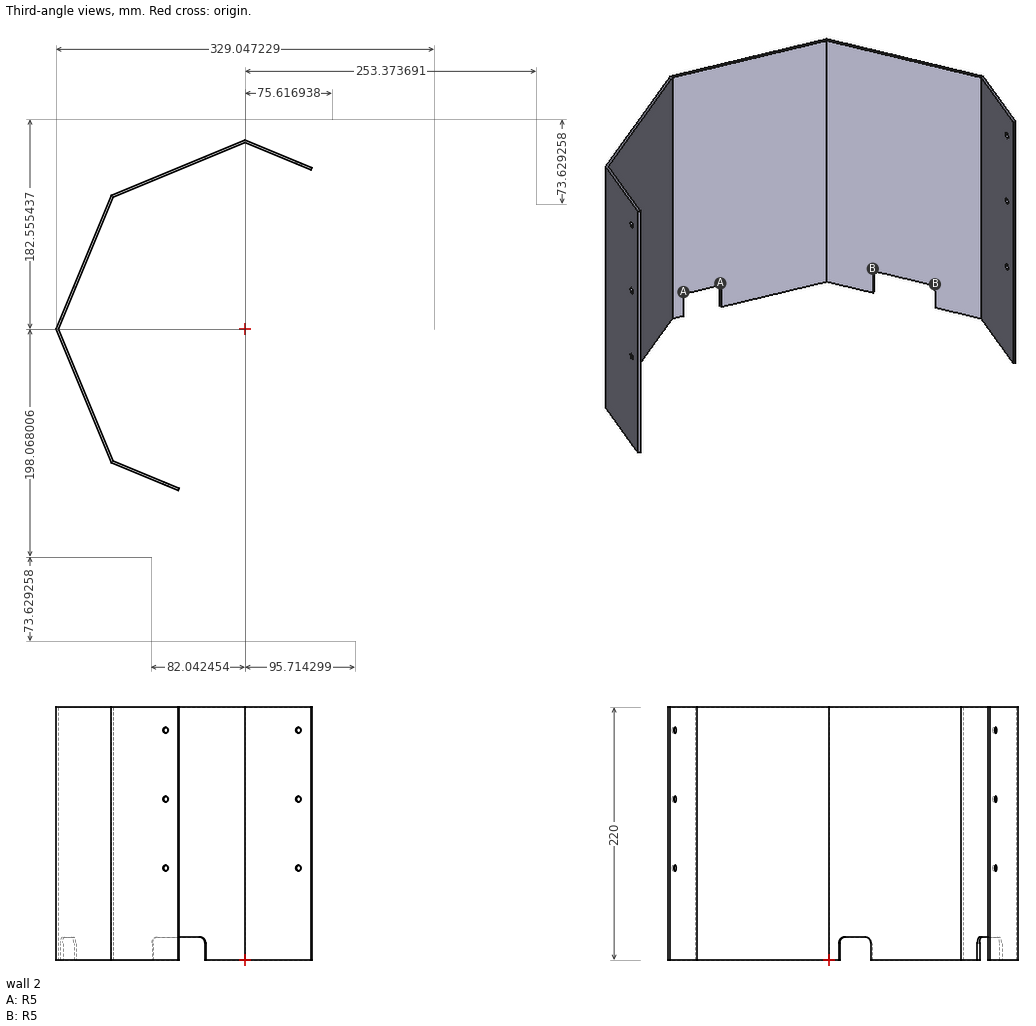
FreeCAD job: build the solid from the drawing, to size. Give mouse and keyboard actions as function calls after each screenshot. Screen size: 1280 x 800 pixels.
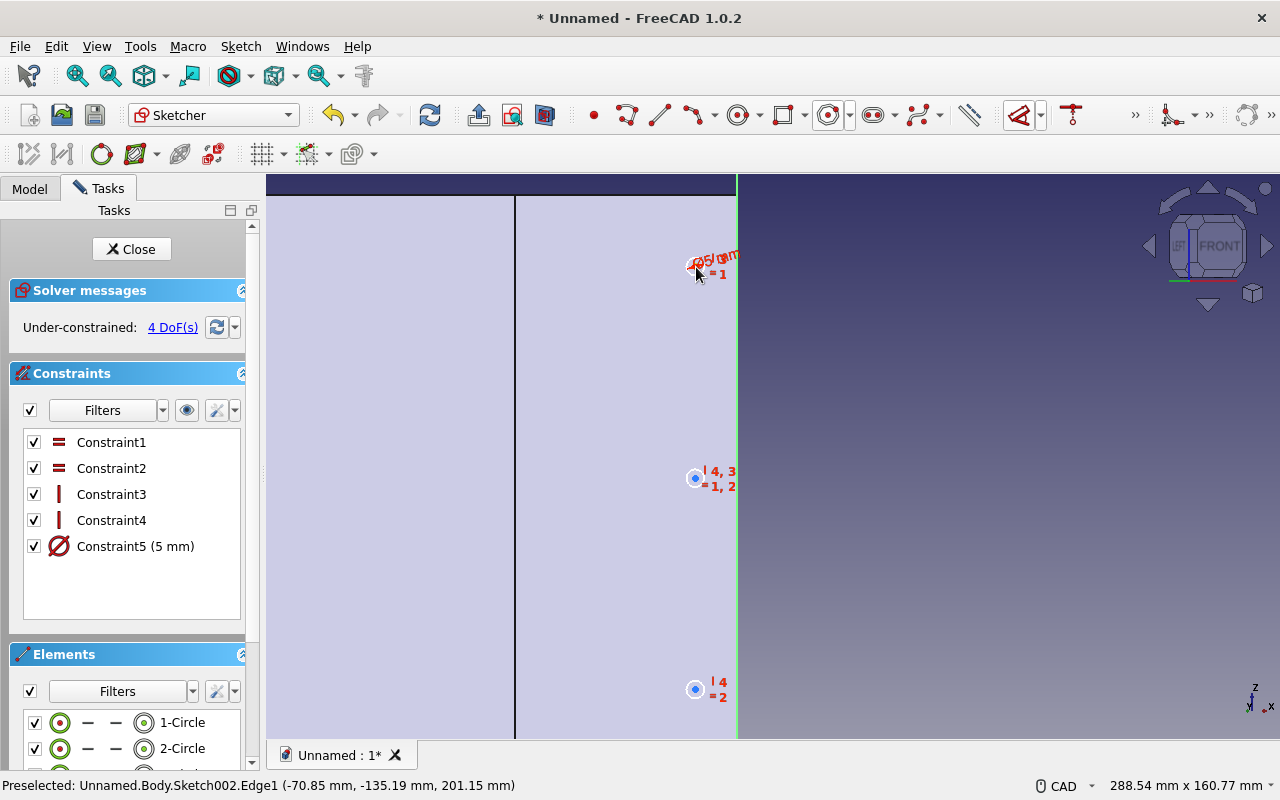
click(695, 267)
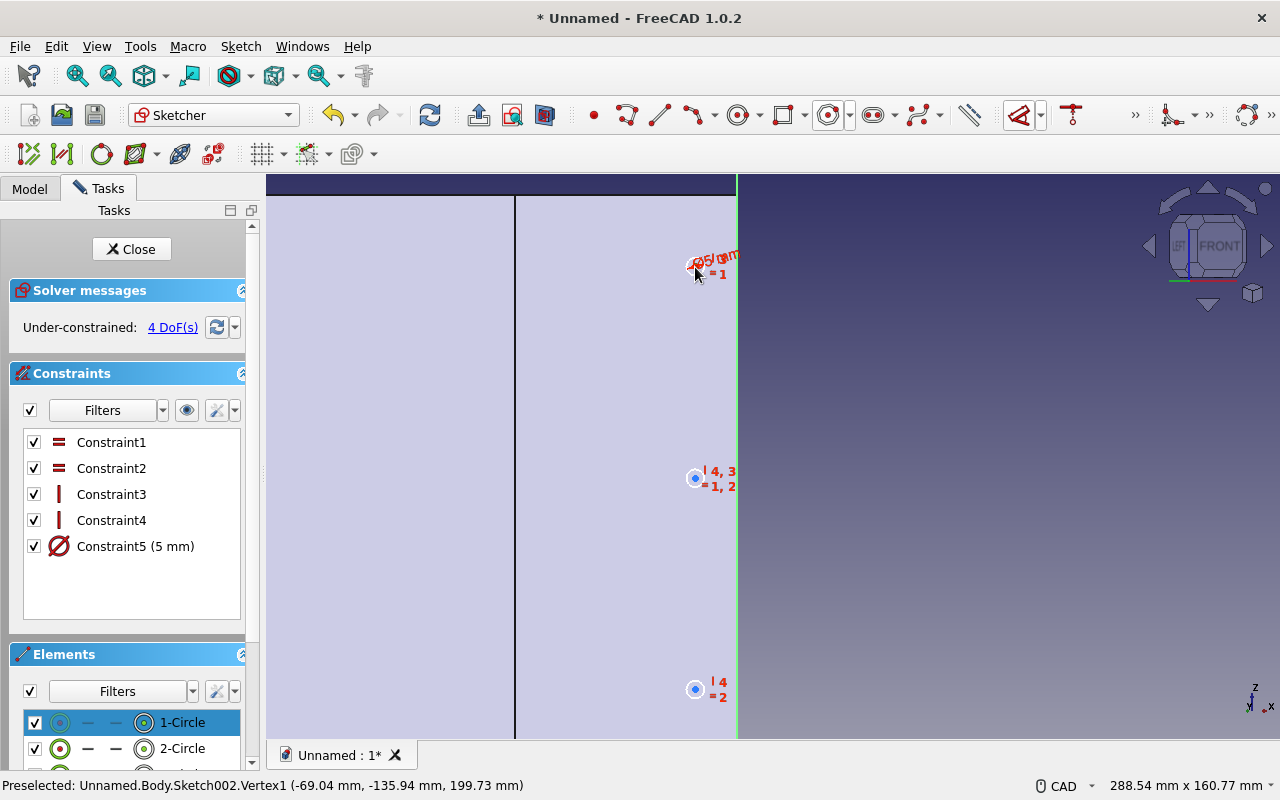
click(1040, 116)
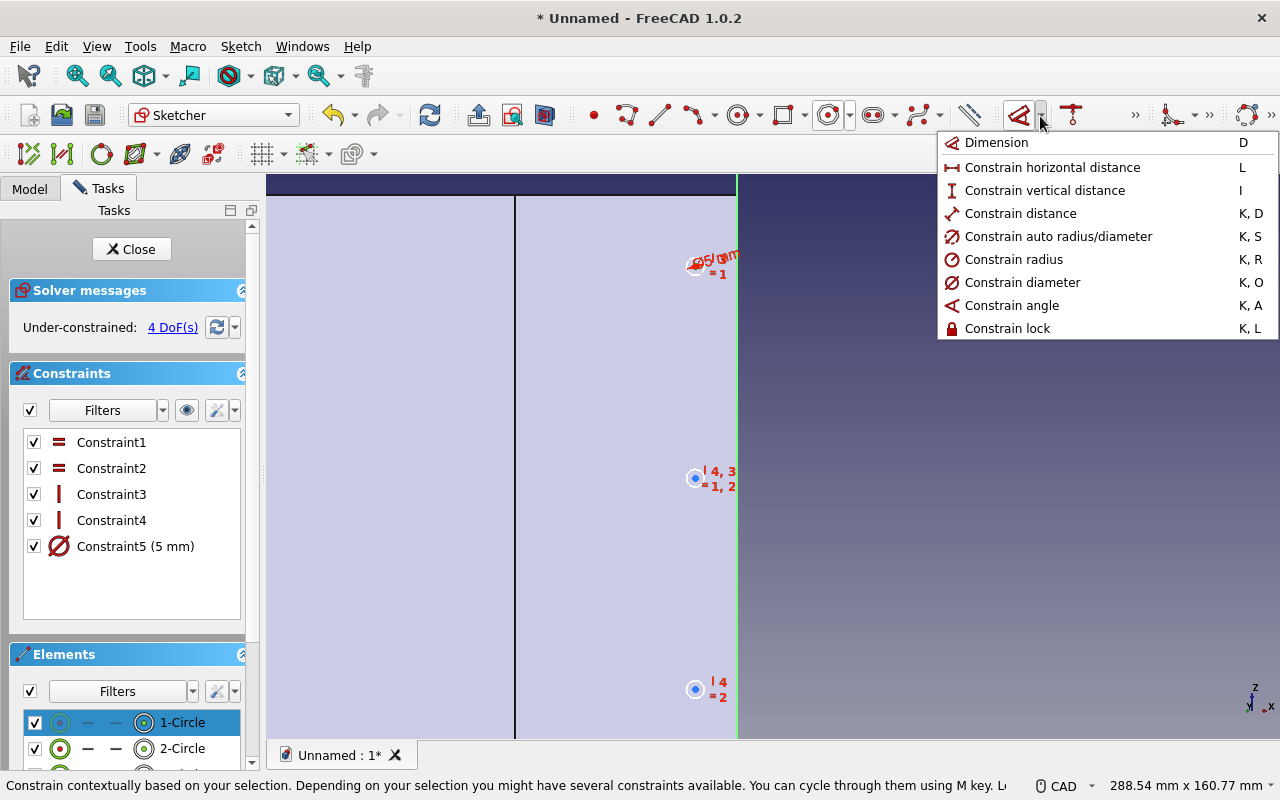
click(1108, 168)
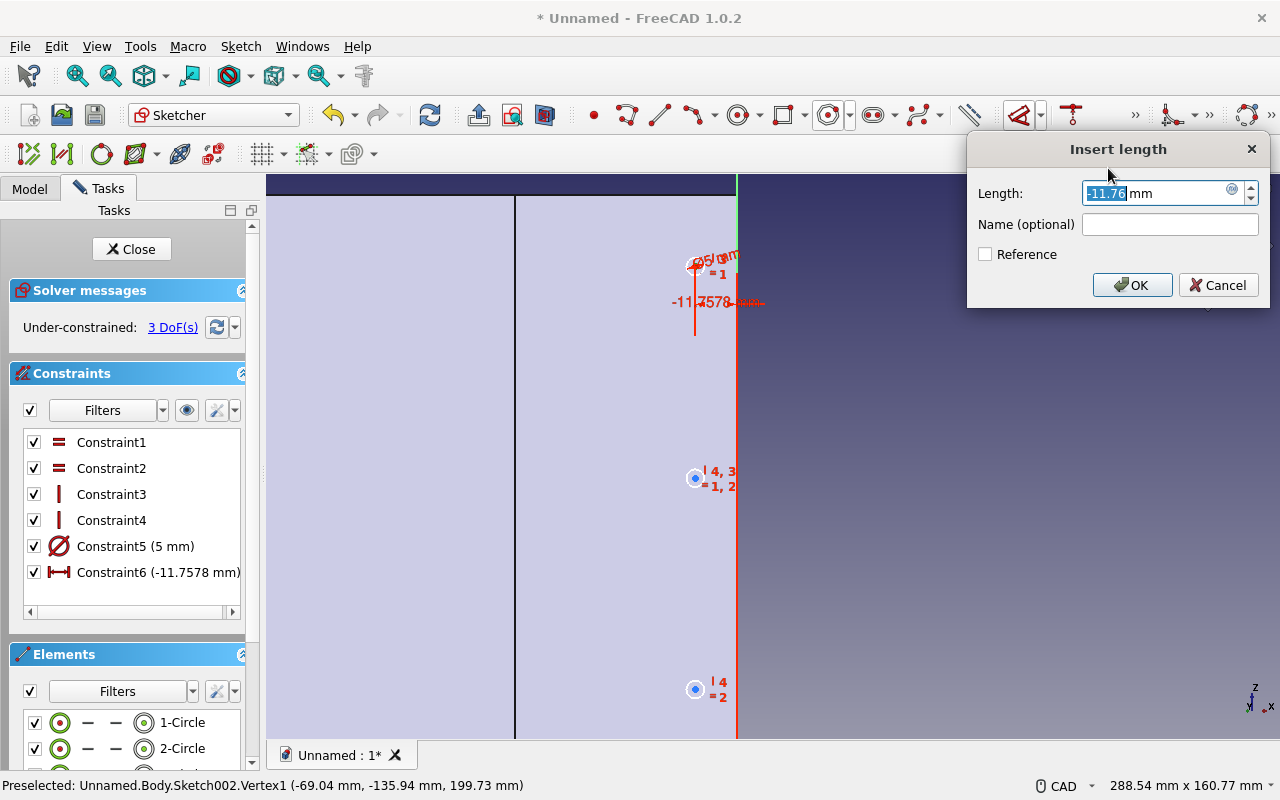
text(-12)
key(Return)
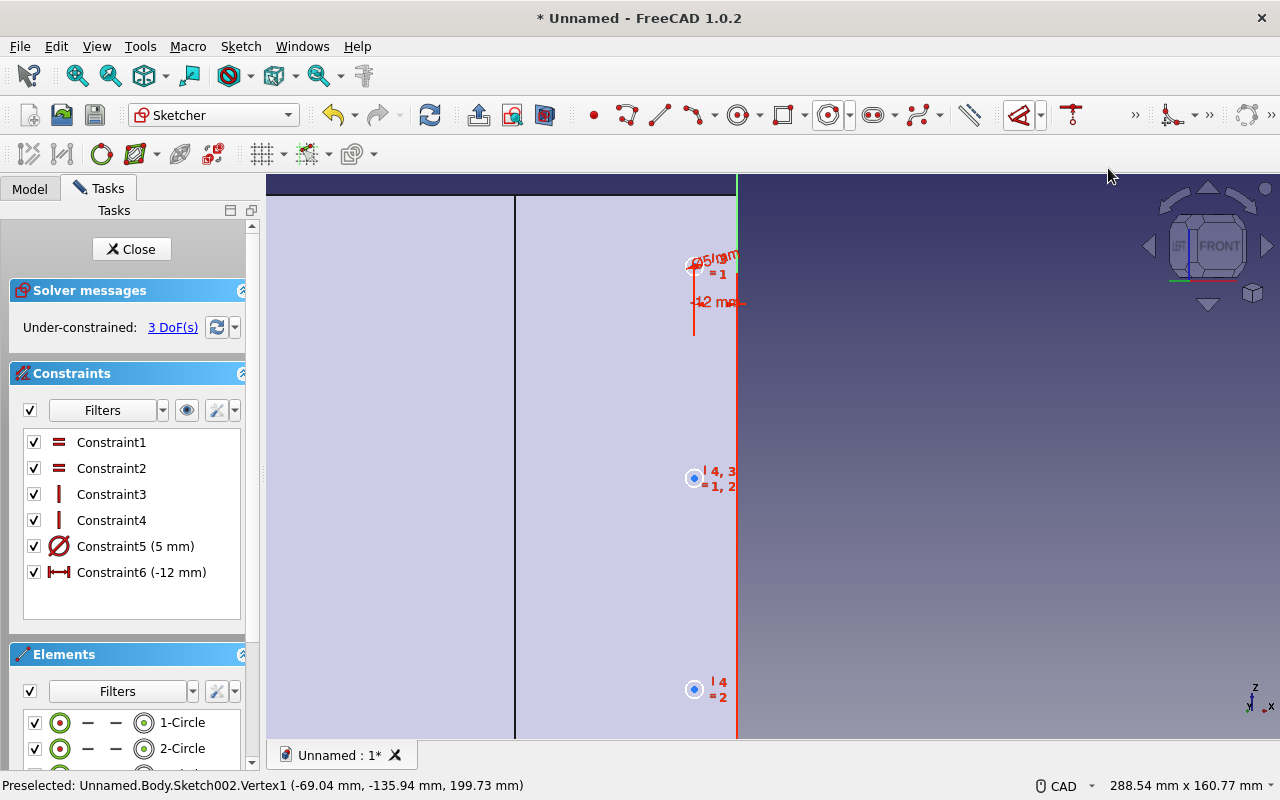
click(694, 690)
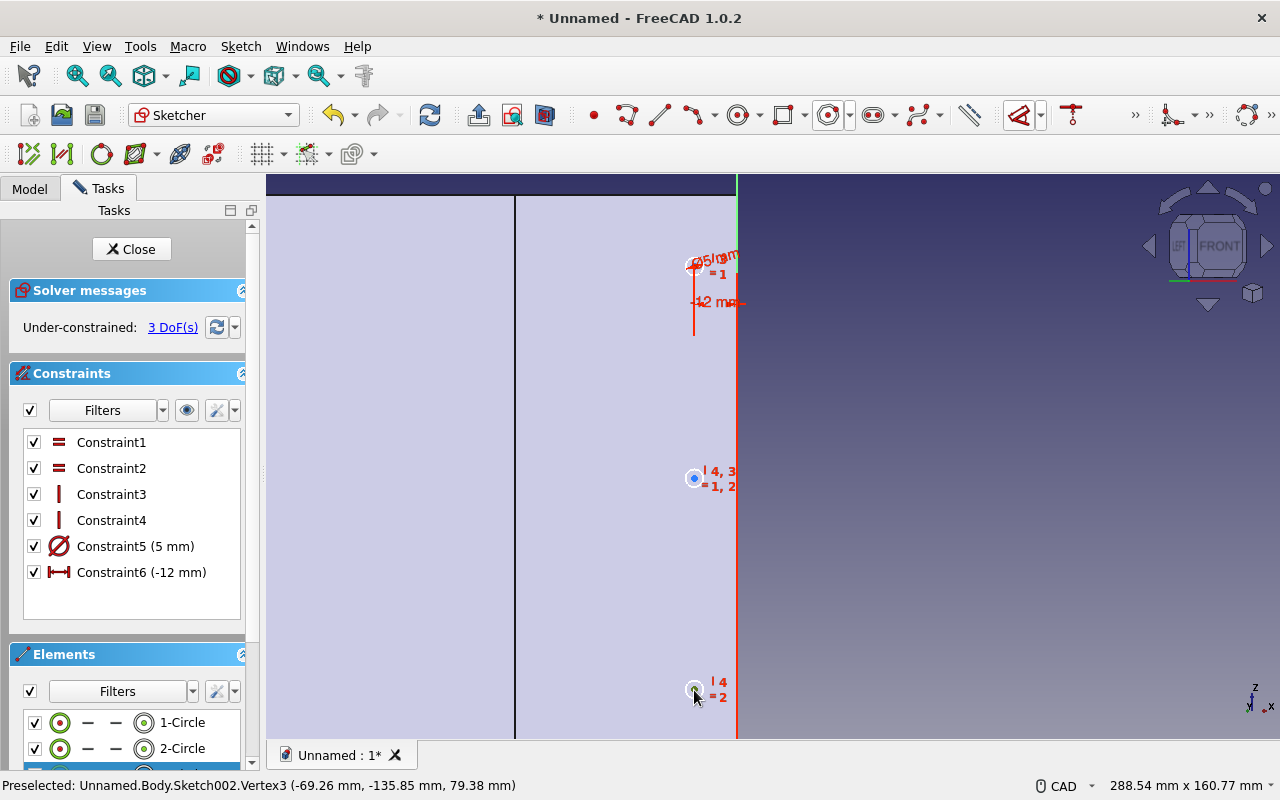
click(1040, 116)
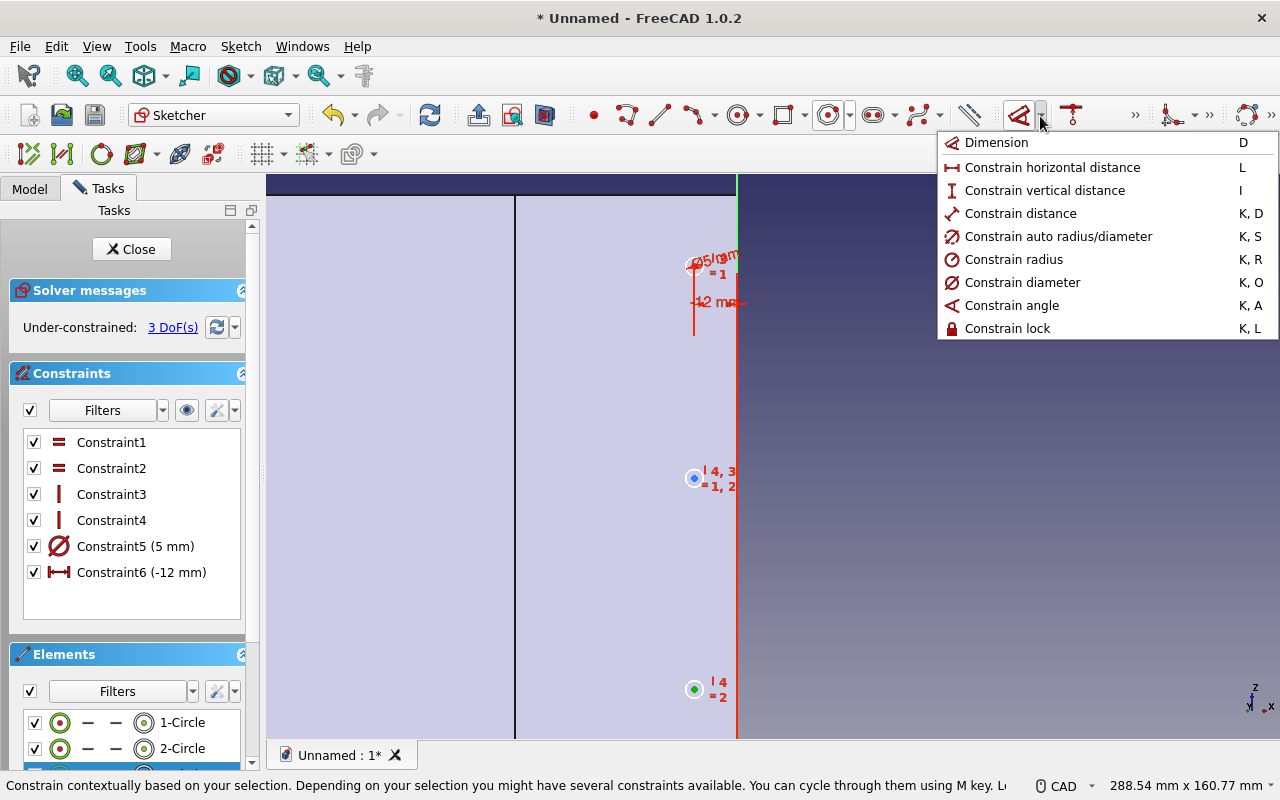
click(1108, 190)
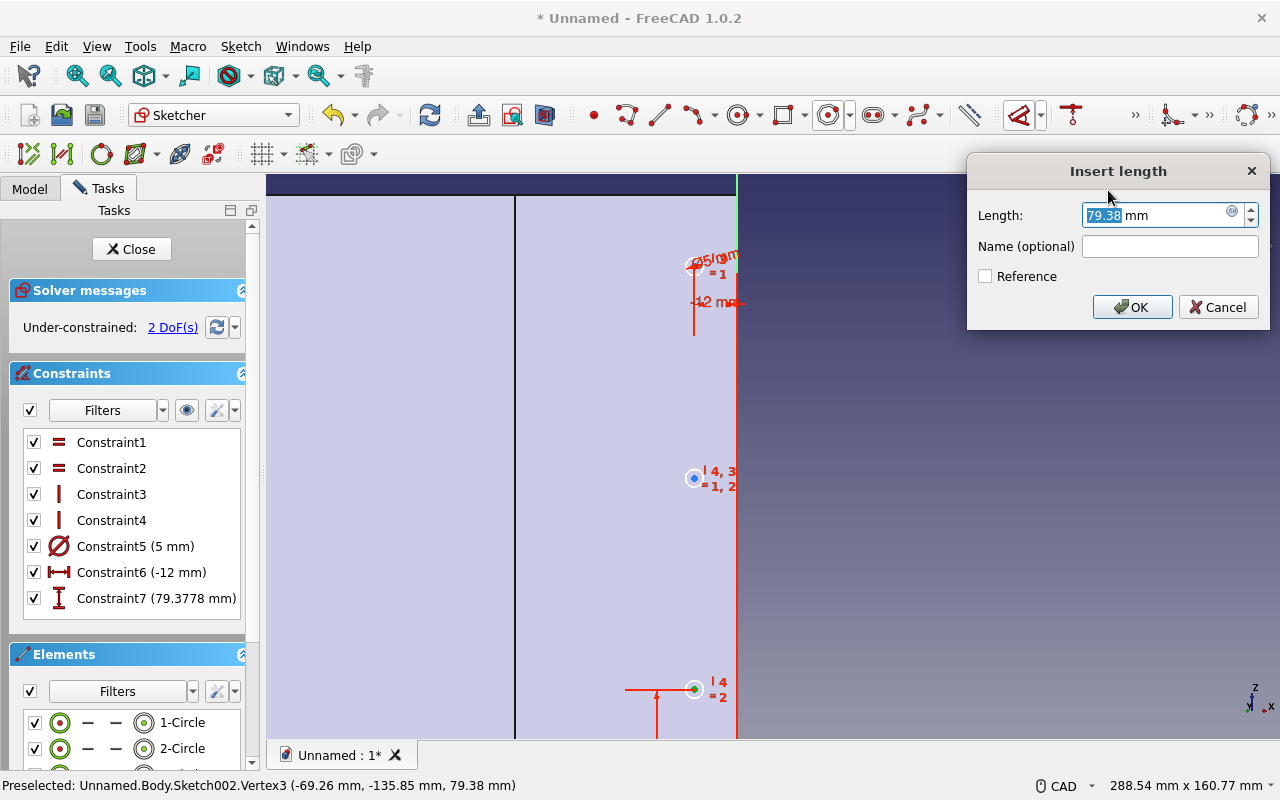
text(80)
key(Return)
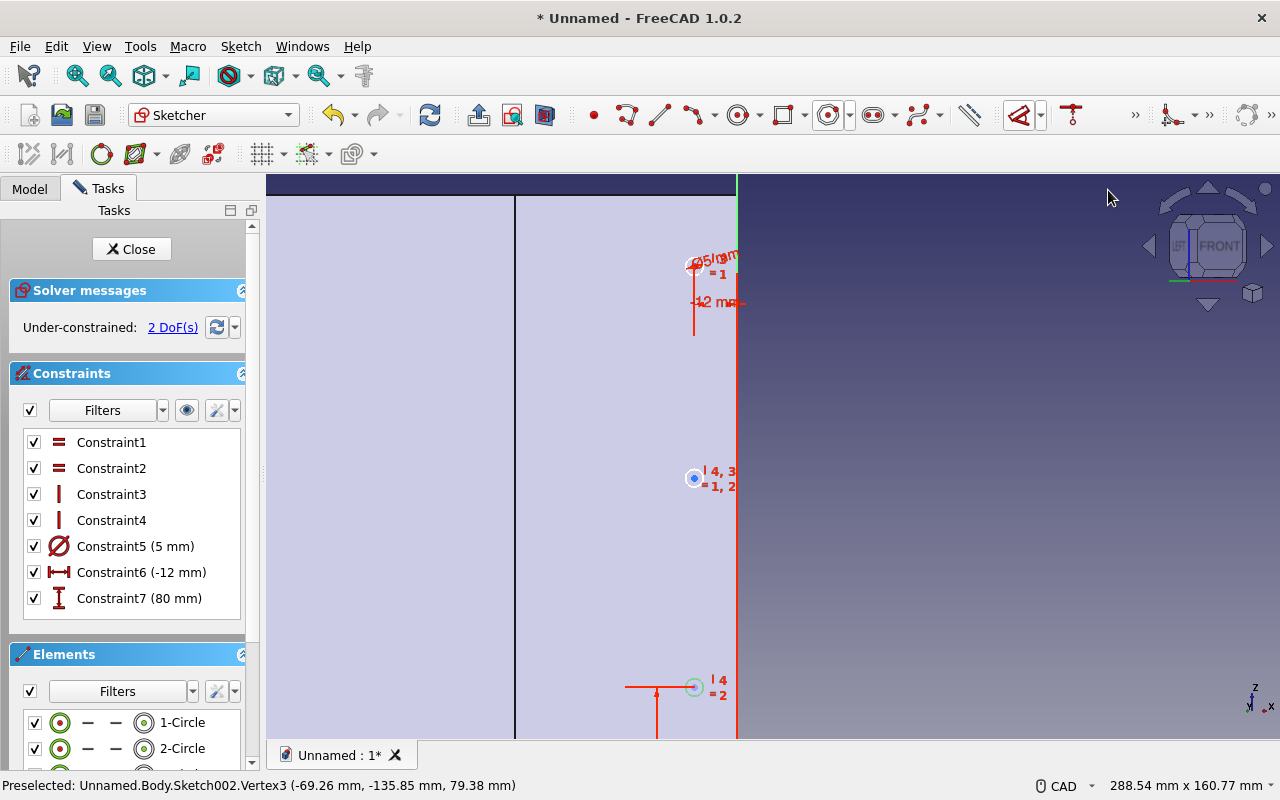
click(694, 267)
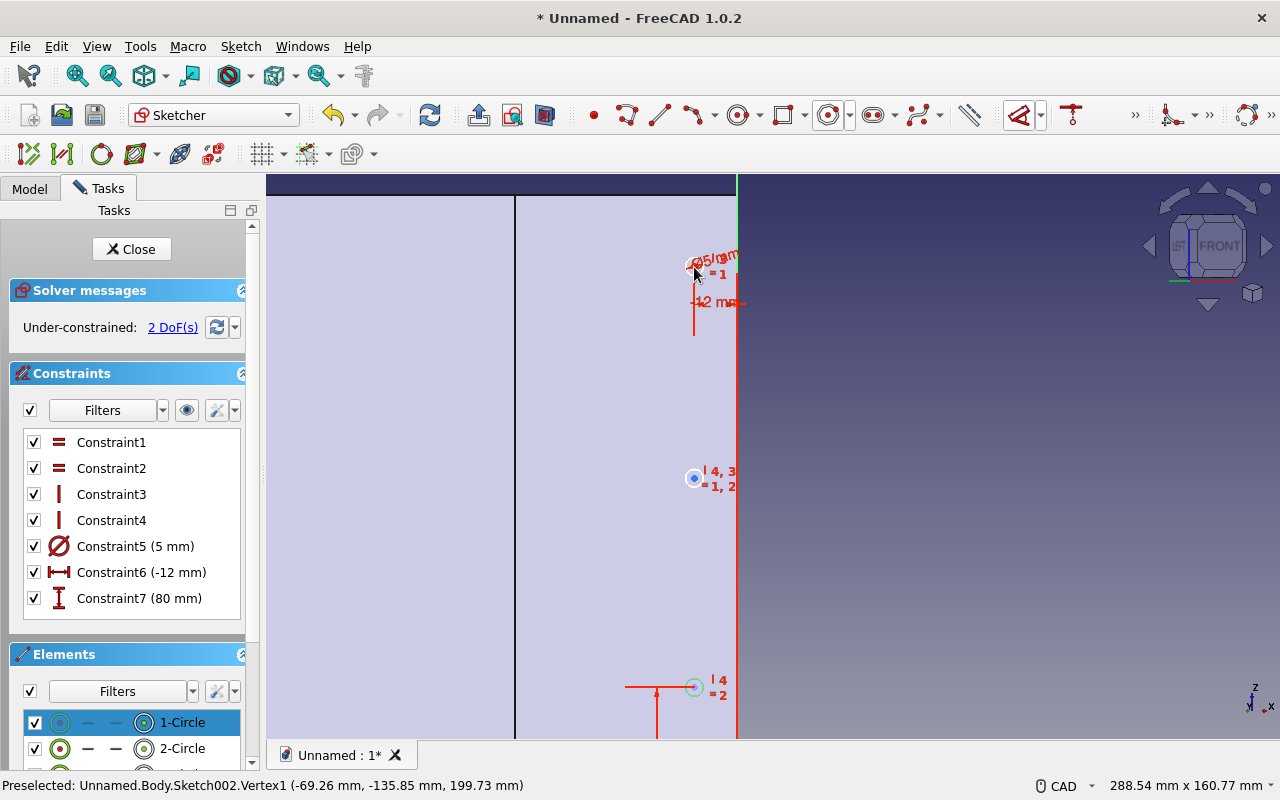
click(1040, 116)